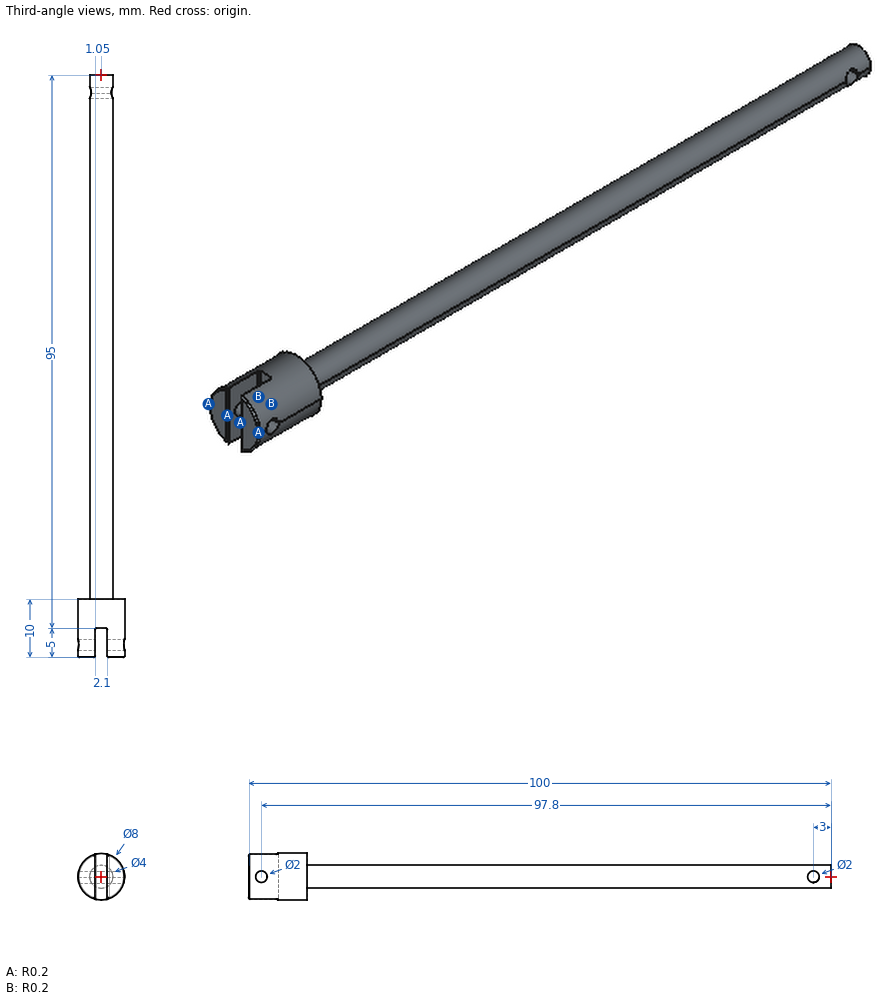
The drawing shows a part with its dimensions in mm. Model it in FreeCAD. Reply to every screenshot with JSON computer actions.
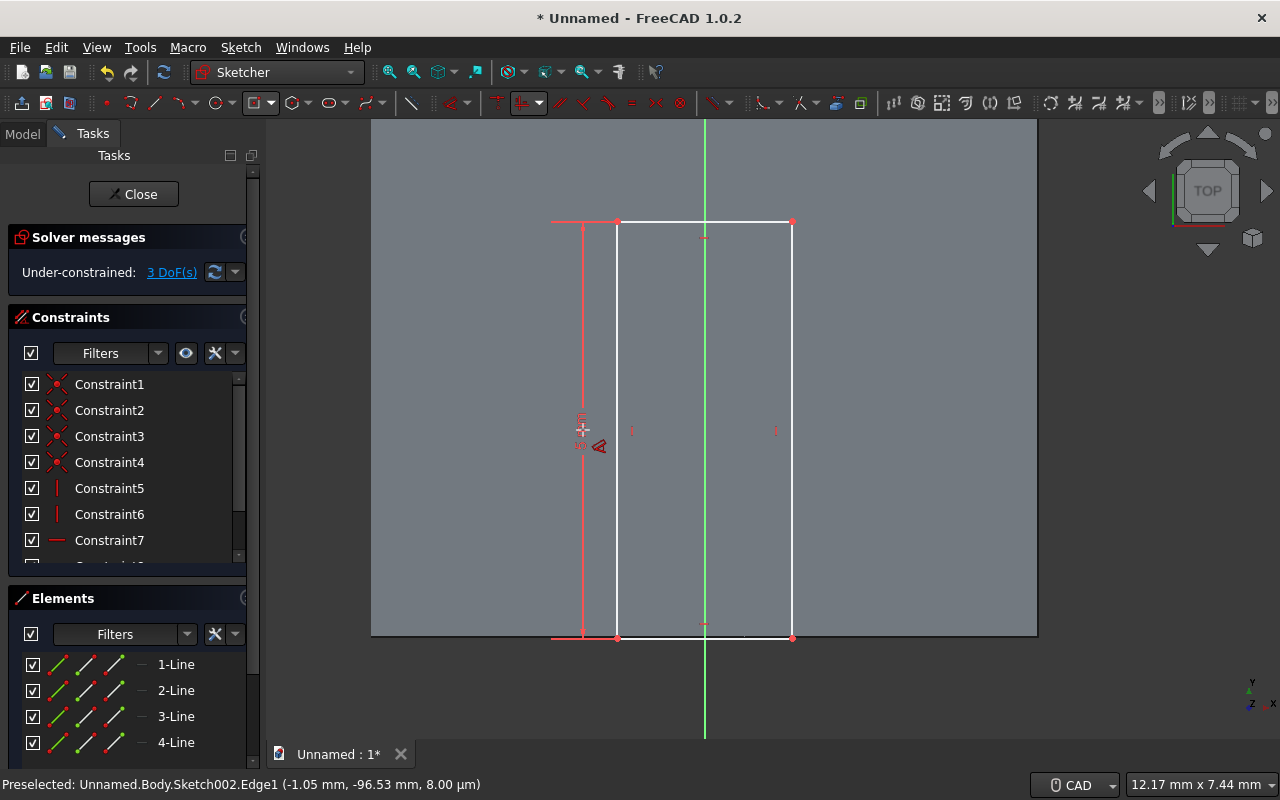
{"action": "left_click", "coordinate": [670, 639]}
{"action": "left_click", "coordinate": [664, 673]}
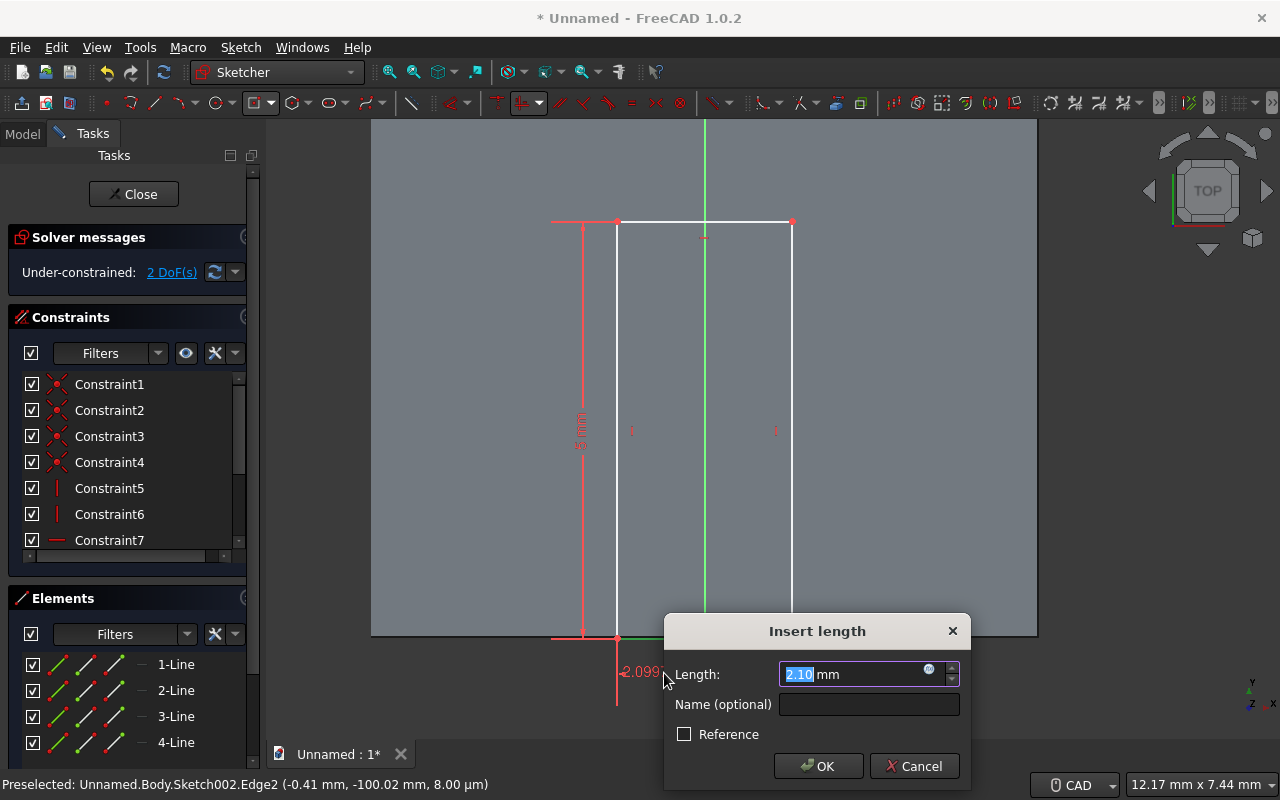
{"action": "type", "text": "2.1"}
{"action": "key", "text": "Return"}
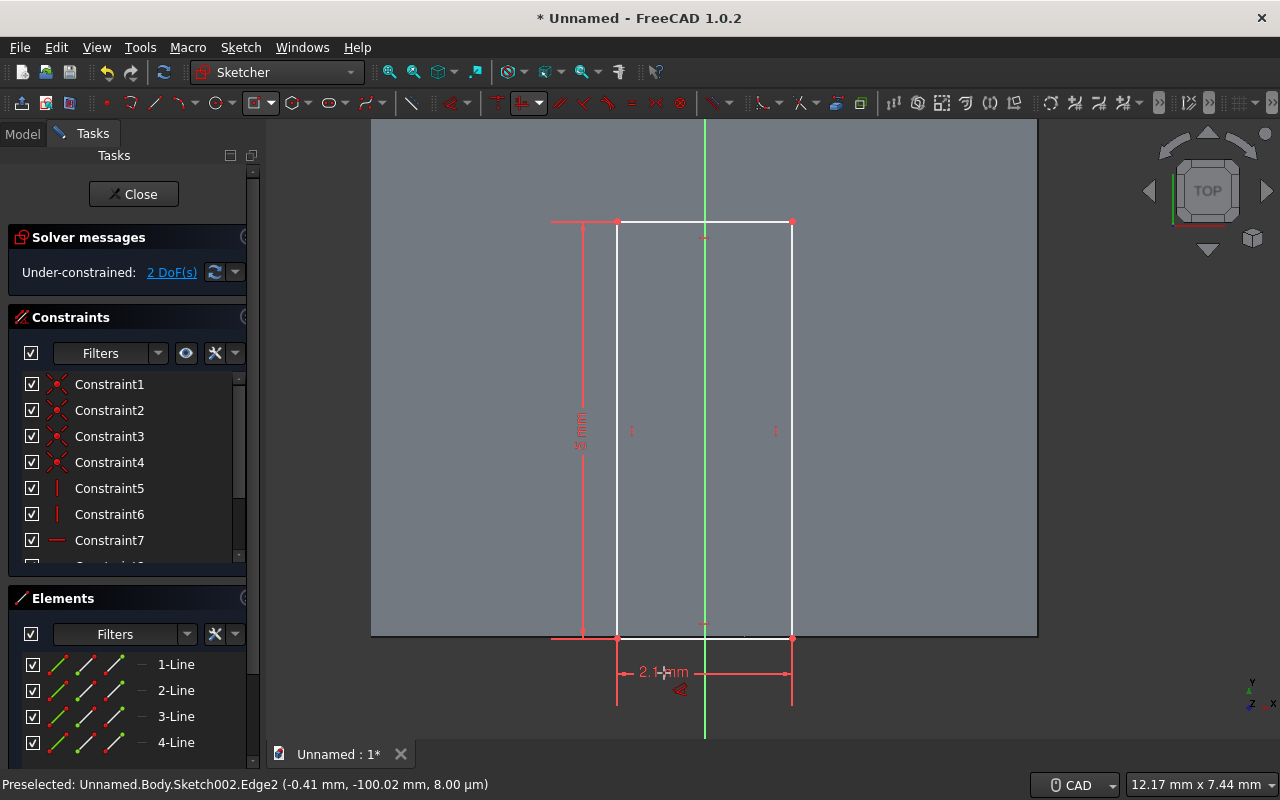
{"action": "left_click", "coordinate": [617, 222]}
{"action": "left_click", "coordinate": [583, 184]}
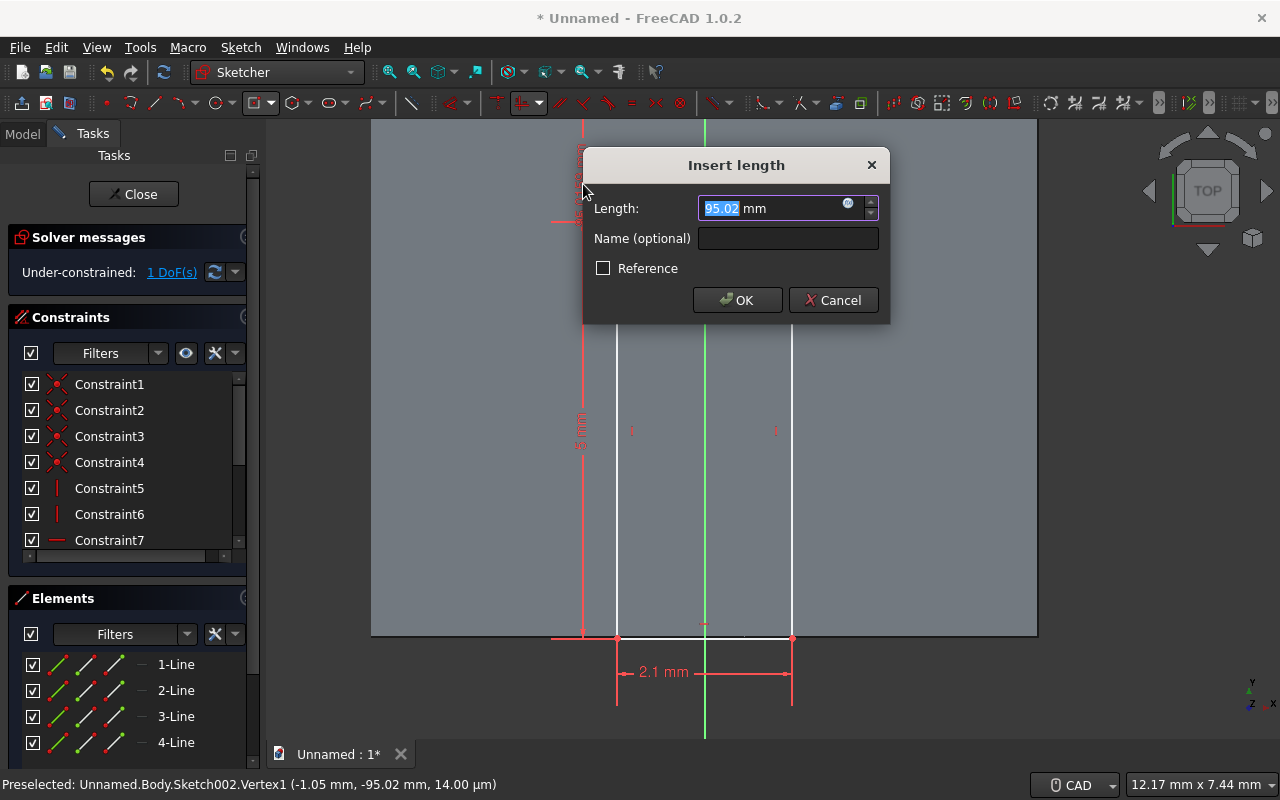
{"action": "type", "text": "95"}
{"action": "key", "text": "Return"}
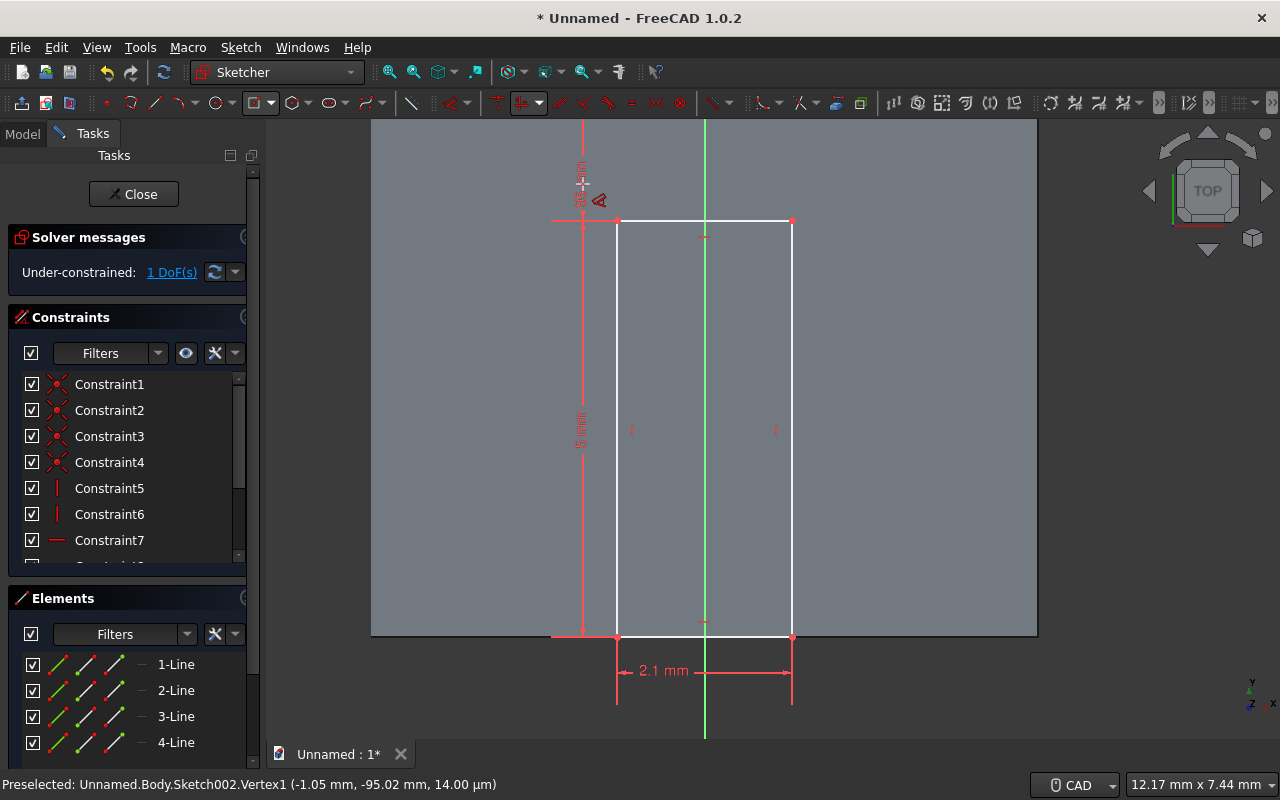
{"action": "left_click", "coordinate": [617, 221]}
{"action": "left_click", "coordinate": [661, 255]}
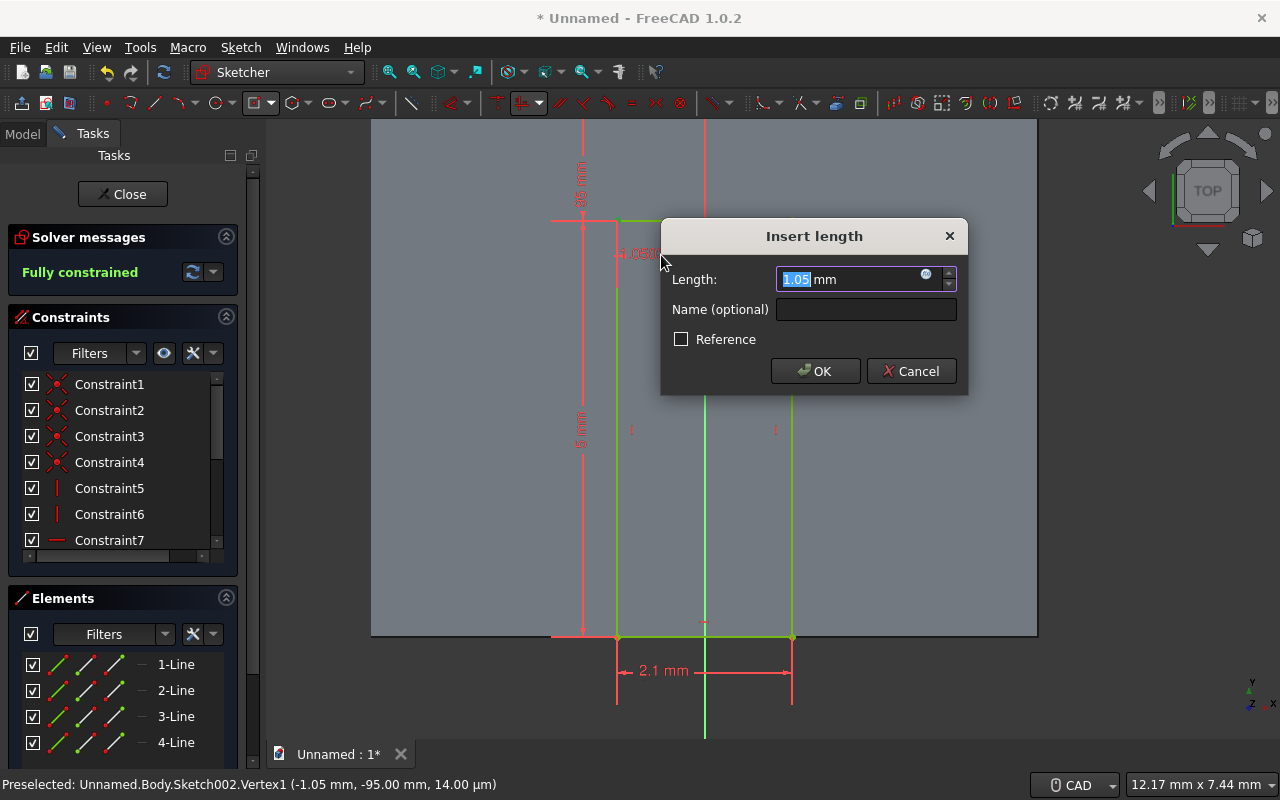
{"action": "type", "text": "1.05"}
{"action": "key", "text": "Return"}
{"action": "key", "text": "Escape"}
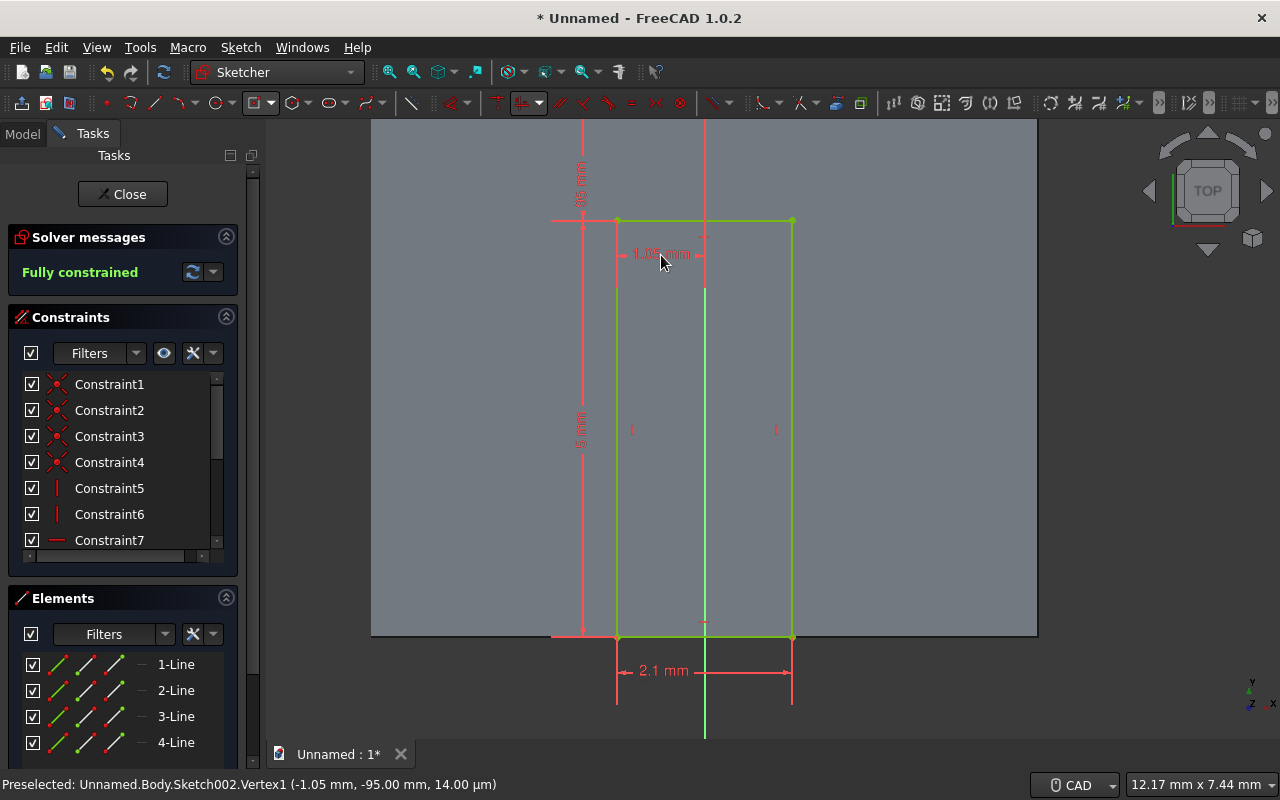
{"action": "left_click", "coordinate": [123, 194]}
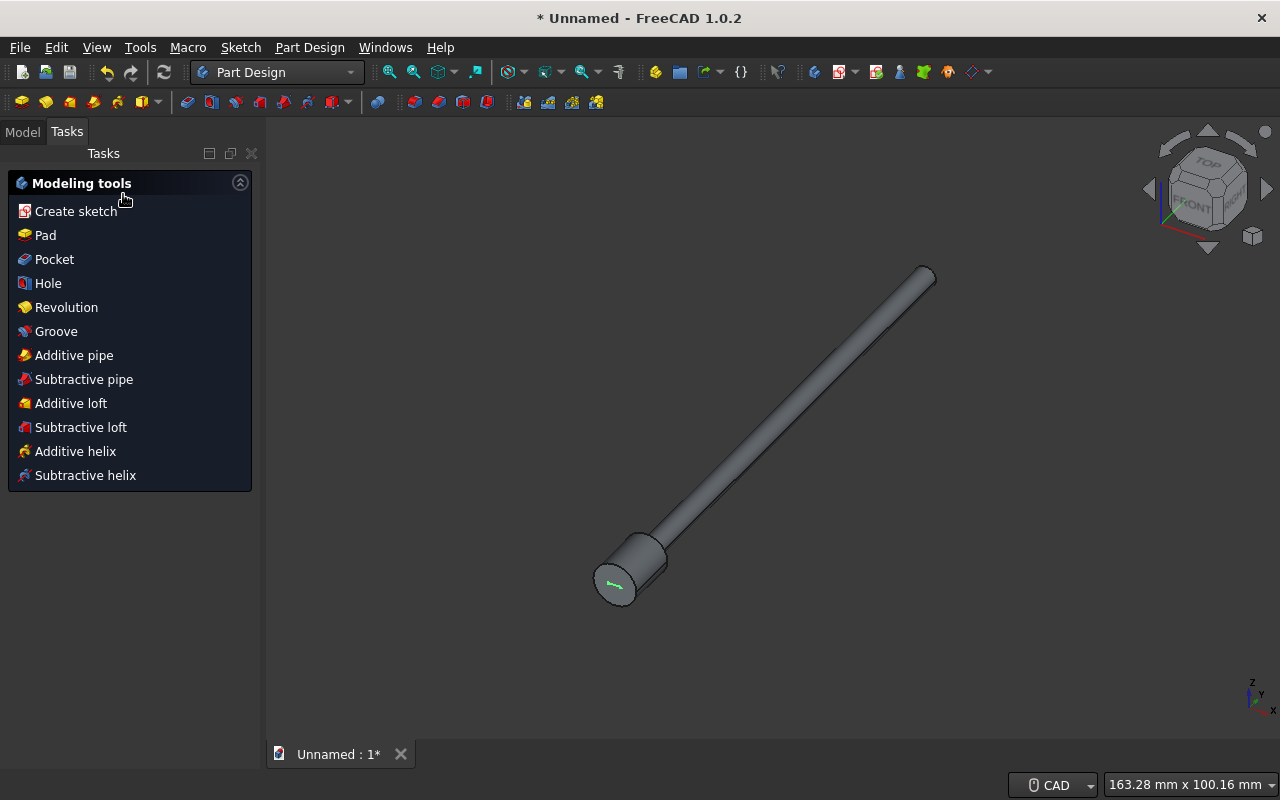
{"action": "left_click", "coordinate": [188, 102]}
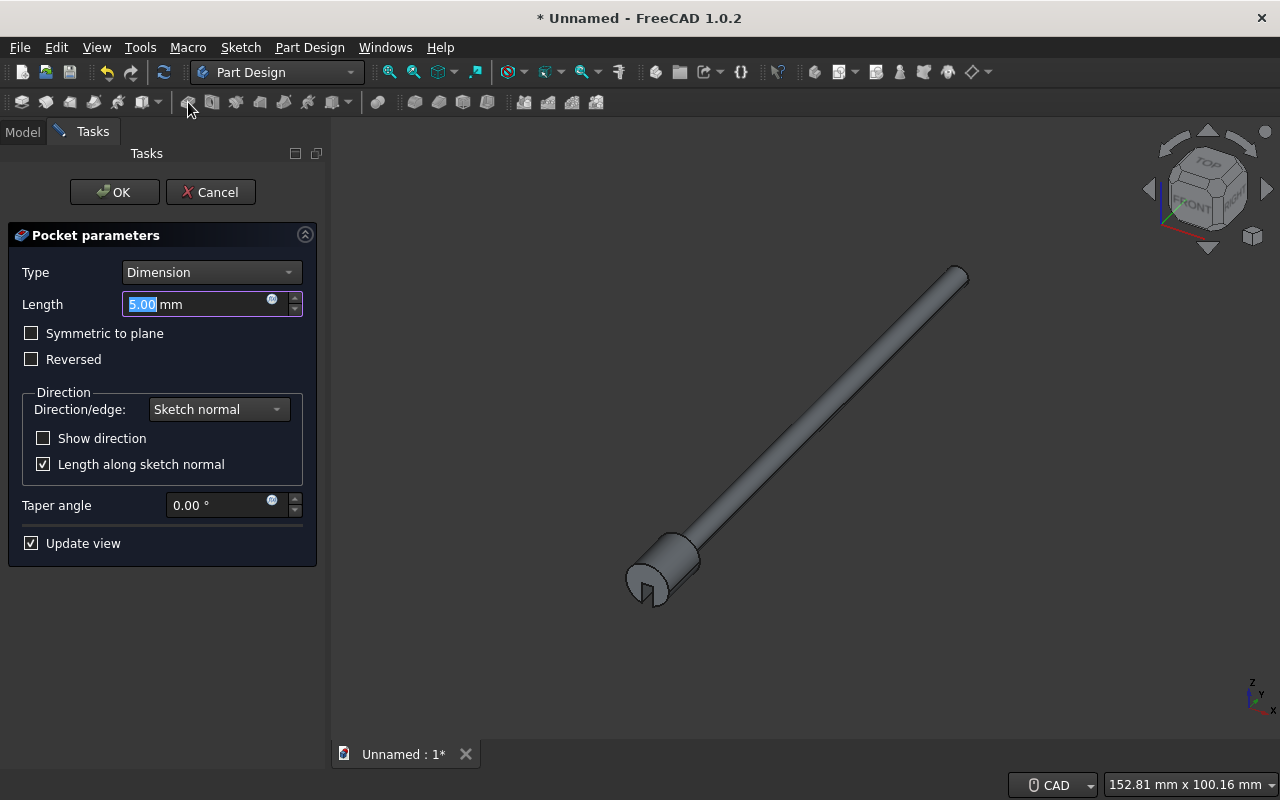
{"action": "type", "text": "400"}
{"action": "key", "text": "Tab"}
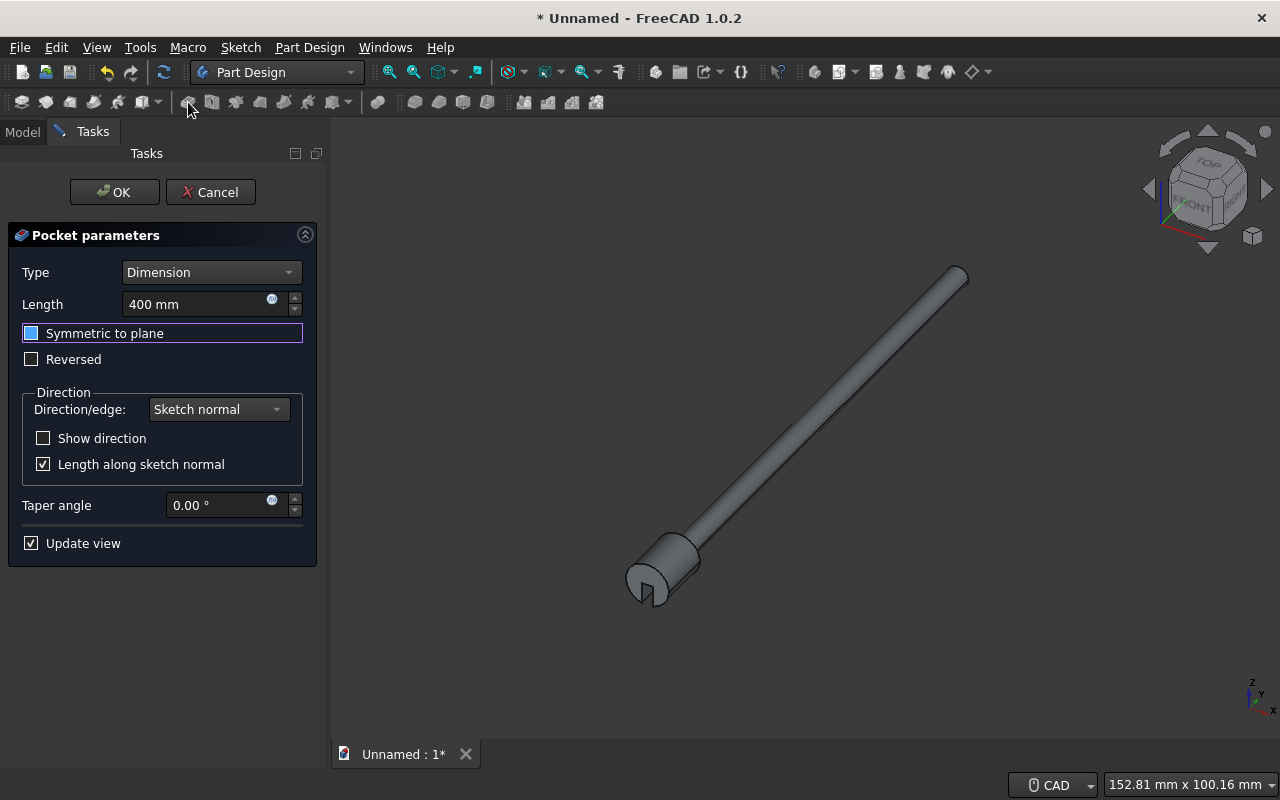
{"action": "left_click", "coordinate": [30, 333]}